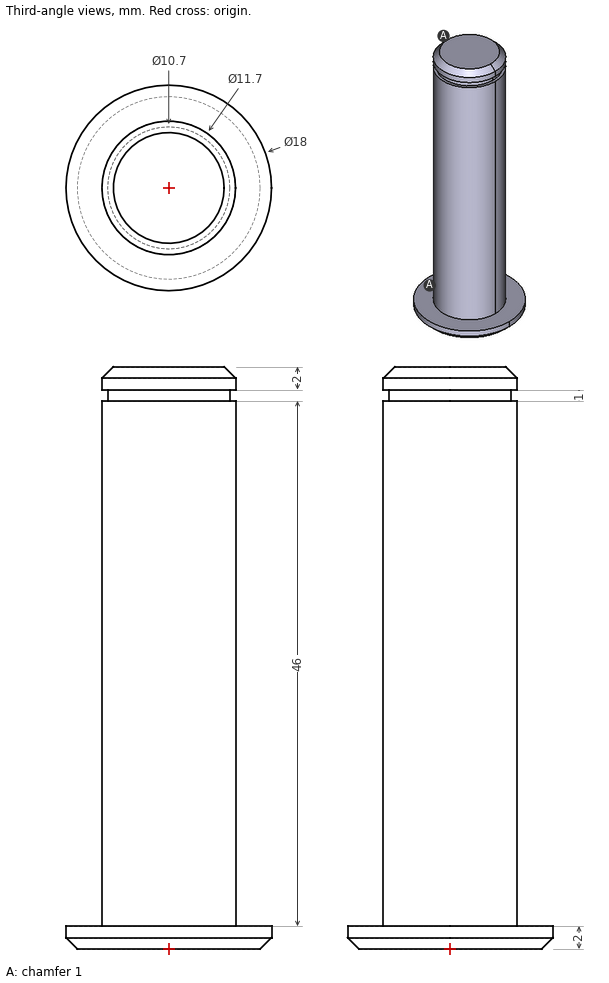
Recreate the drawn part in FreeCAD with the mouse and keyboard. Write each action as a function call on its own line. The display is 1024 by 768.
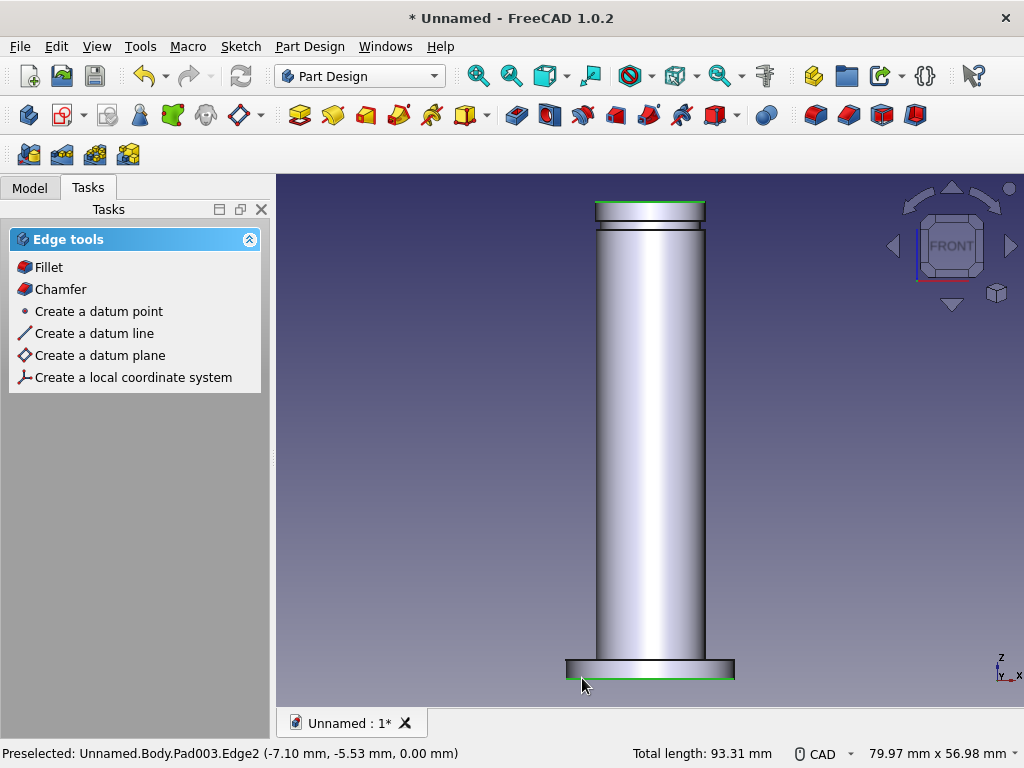
click(849, 116)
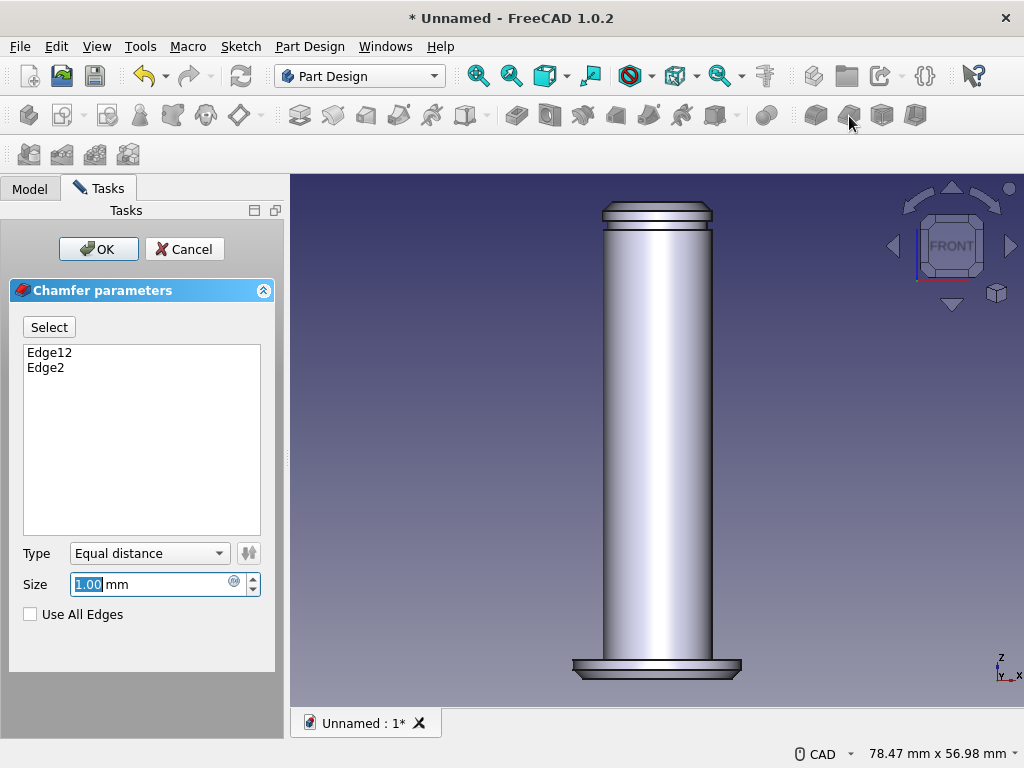
text(1)
key(Tab)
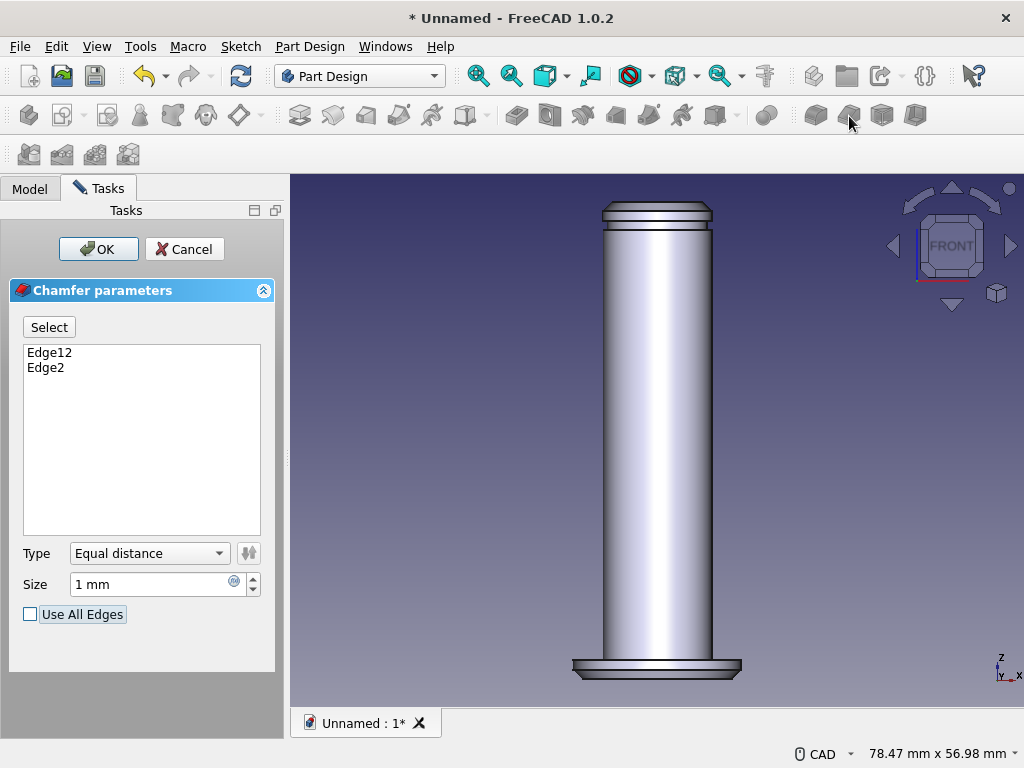
click(99, 249)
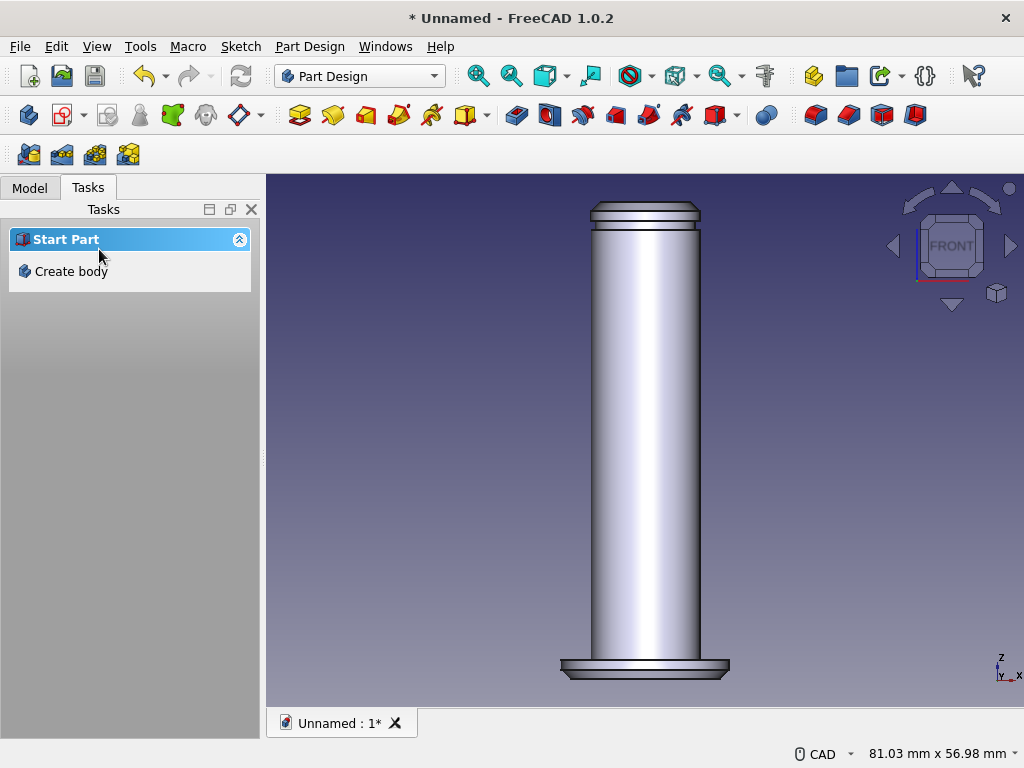
key(0)